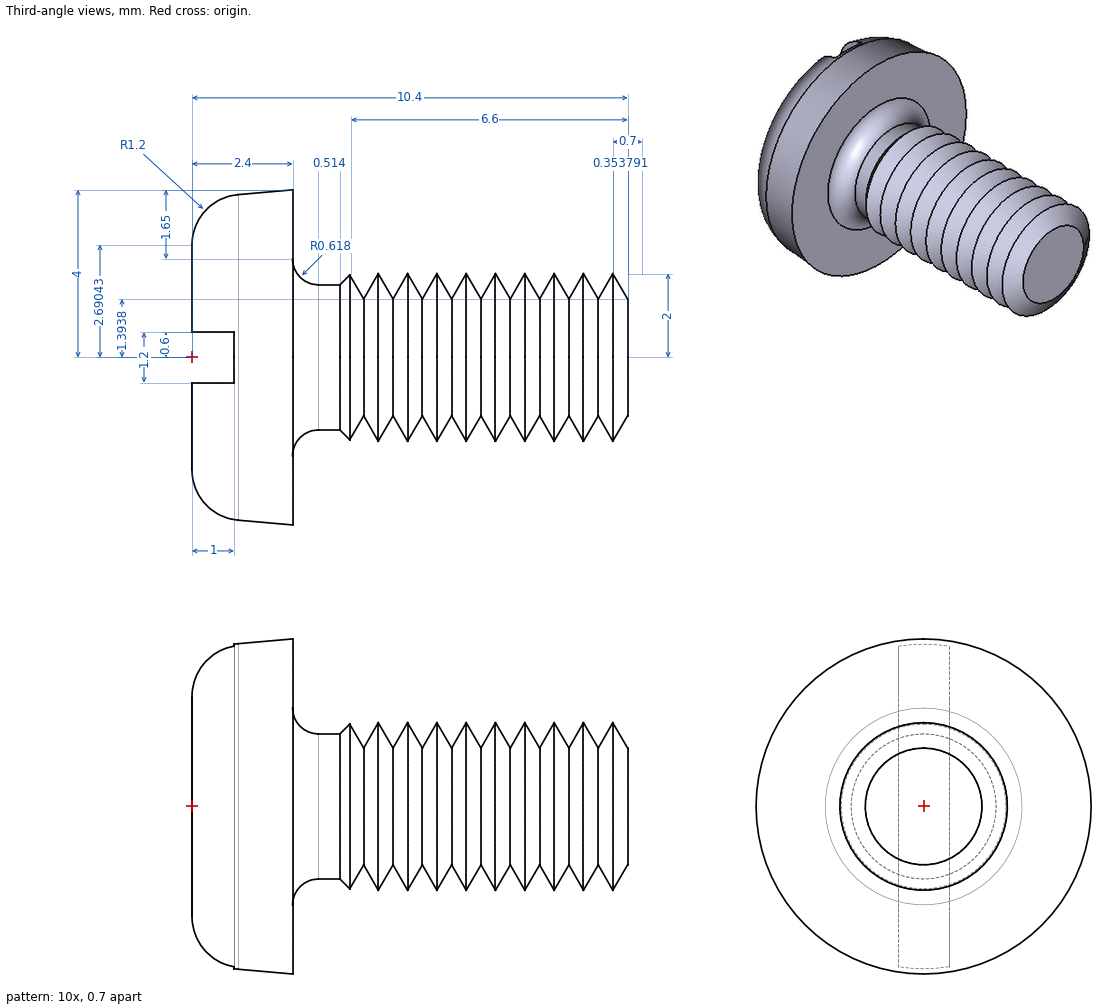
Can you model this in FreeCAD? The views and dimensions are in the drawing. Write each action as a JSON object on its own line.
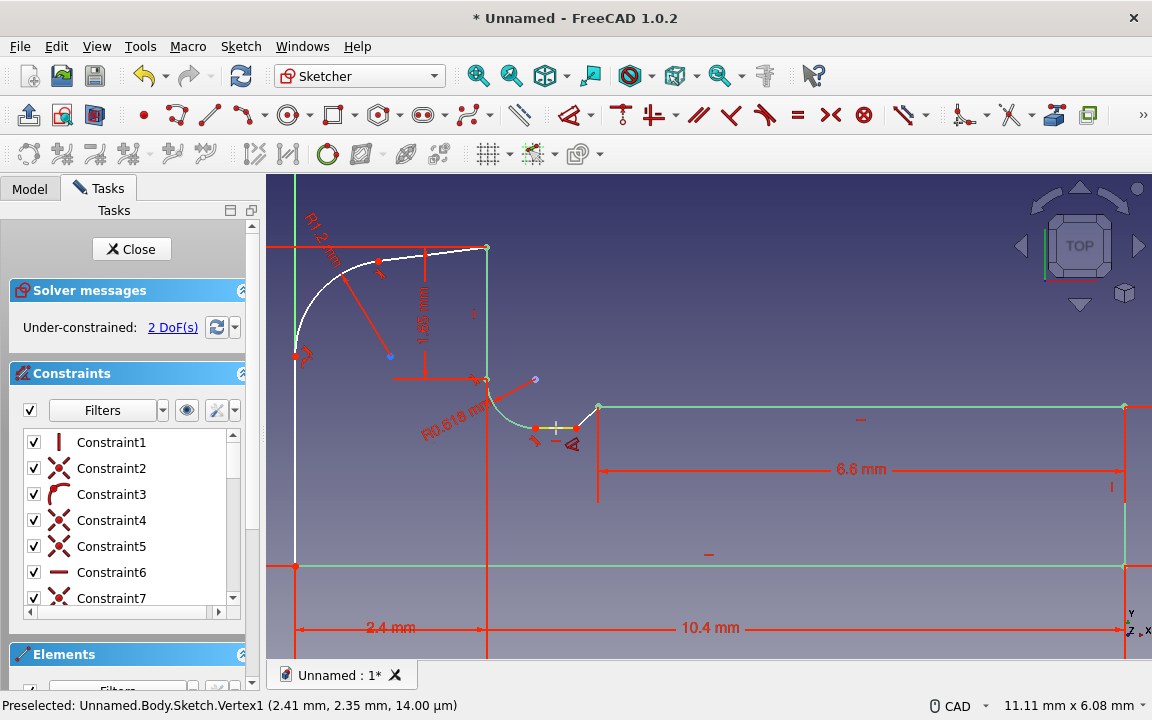
{"action": "left_click", "coordinate": [556, 428]}
{"action": "left_click", "coordinate": [556, 462]}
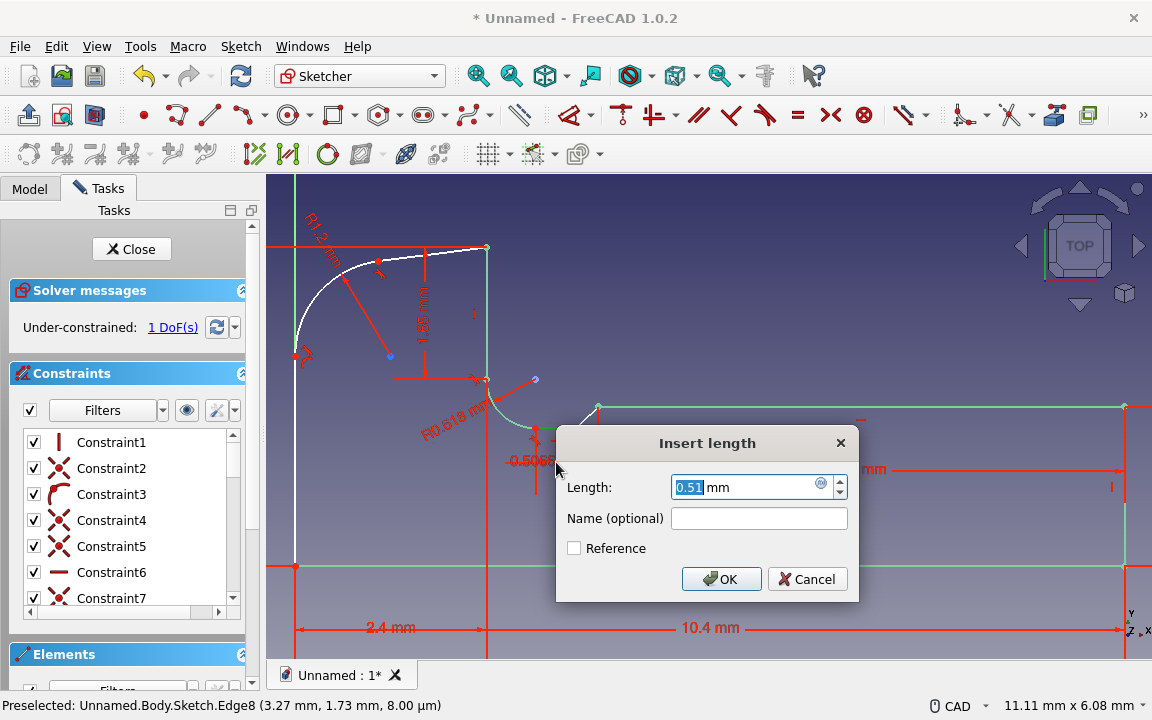
{"action": "type", "text": "0.514"}
{"action": "key", "text": "Return"}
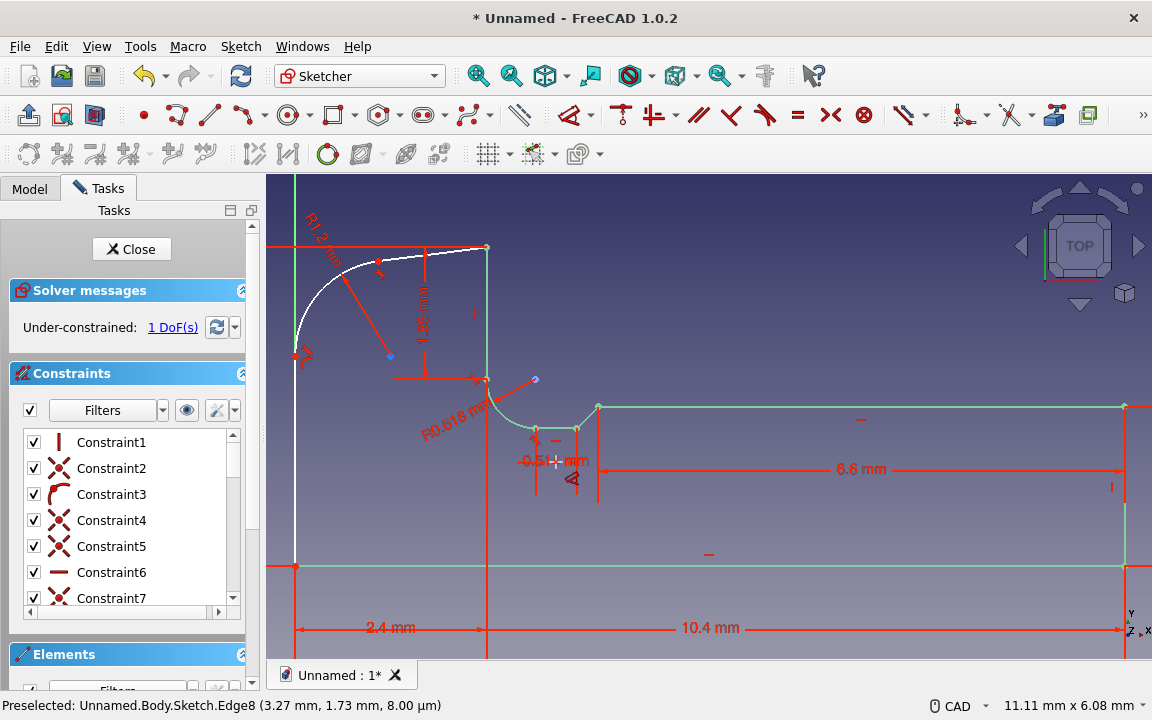
{"action": "left_click", "coordinate": [295, 419]}
{"action": "left_click", "coordinate": [329, 461]}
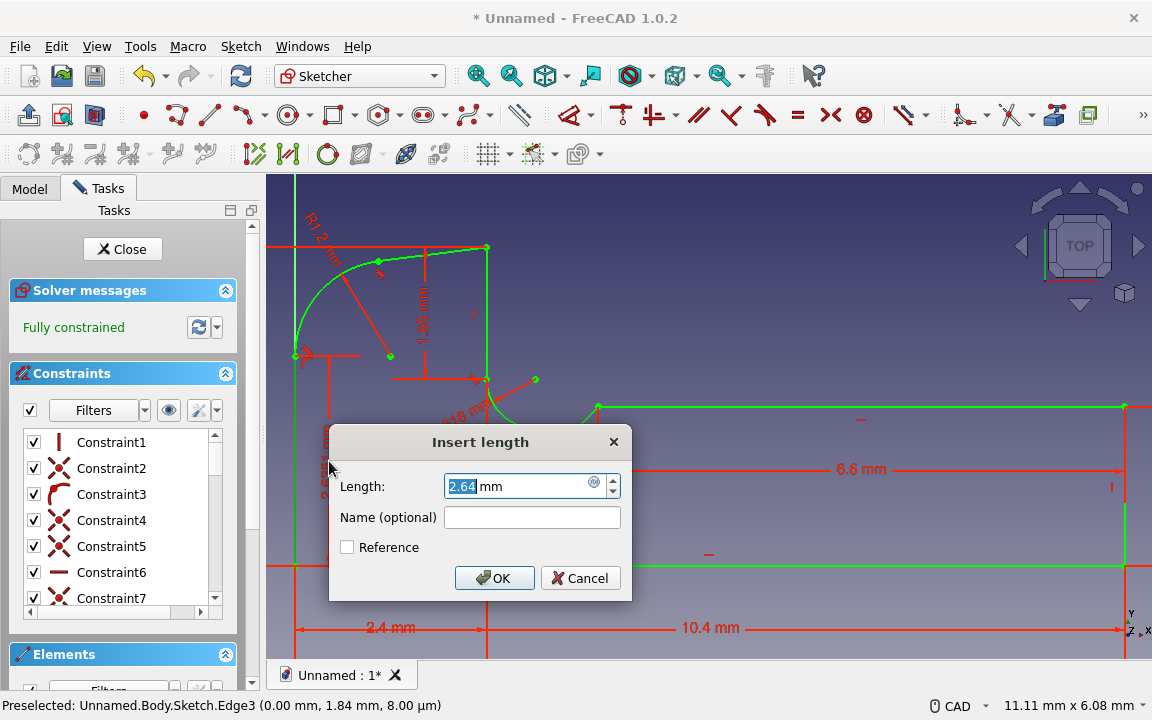
{"action": "type", "text": "2.69043"}
{"action": "key", "text": "Return"}
{"action": "key", "text": "Escape"}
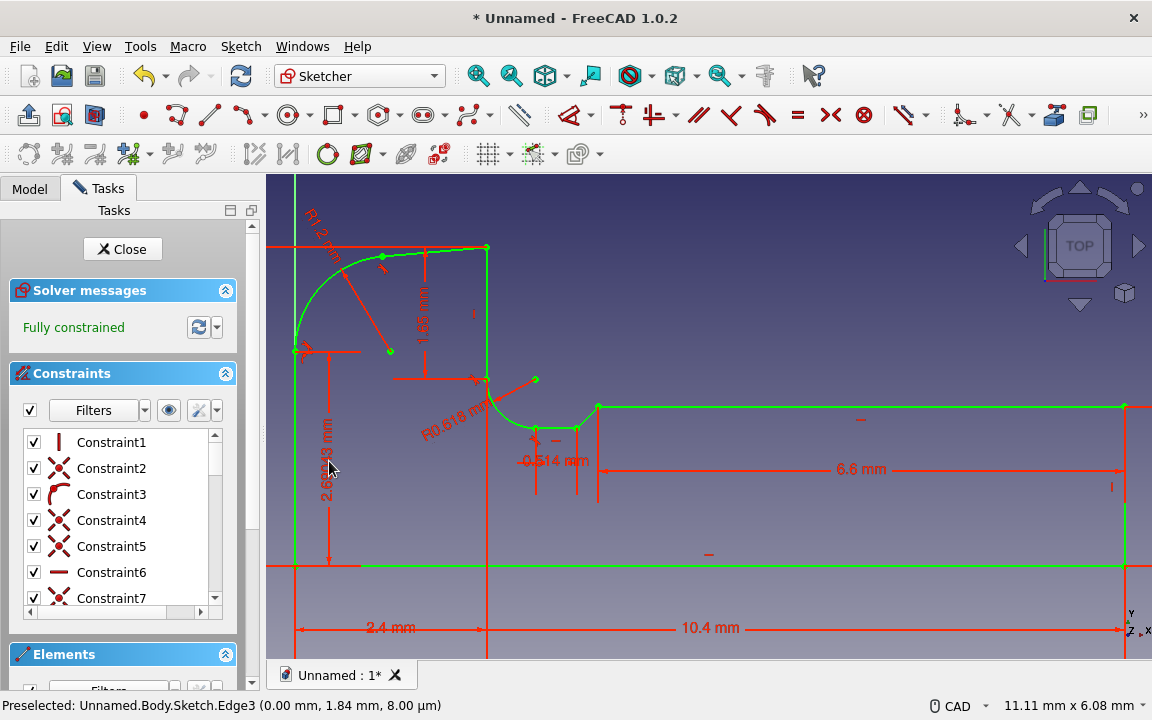
{"action": "left_click", "coordinate": [123, 249]}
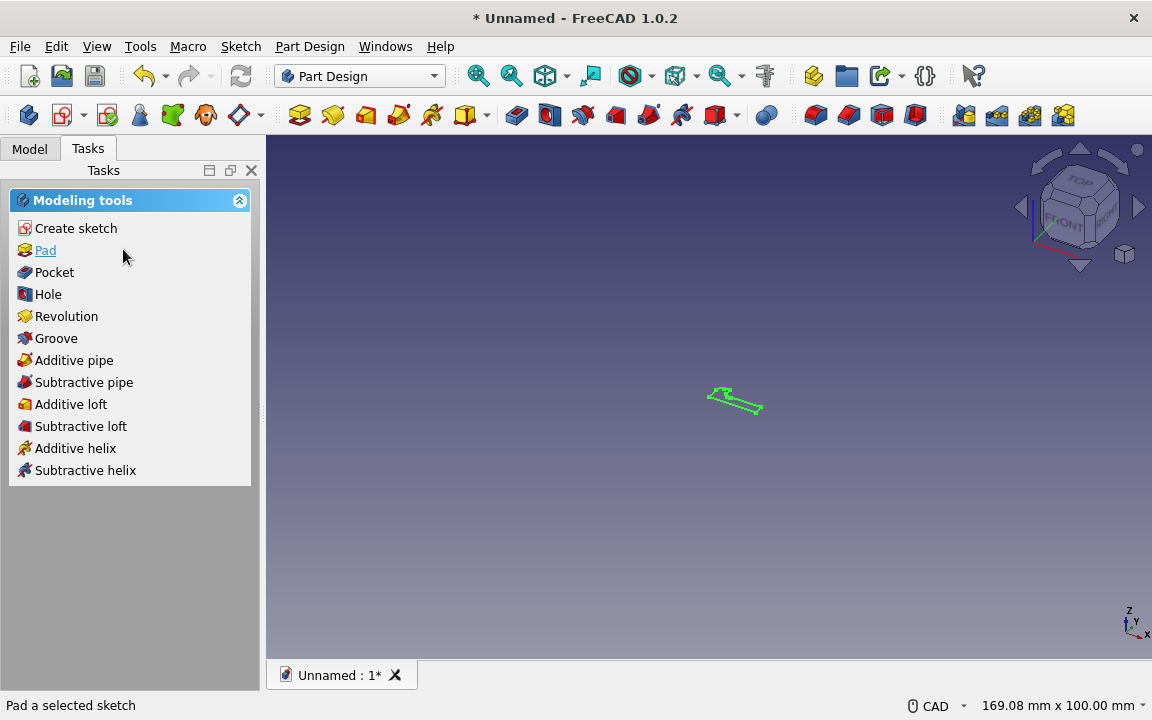
{"action": "left_click", "coordinate": [333, 116]}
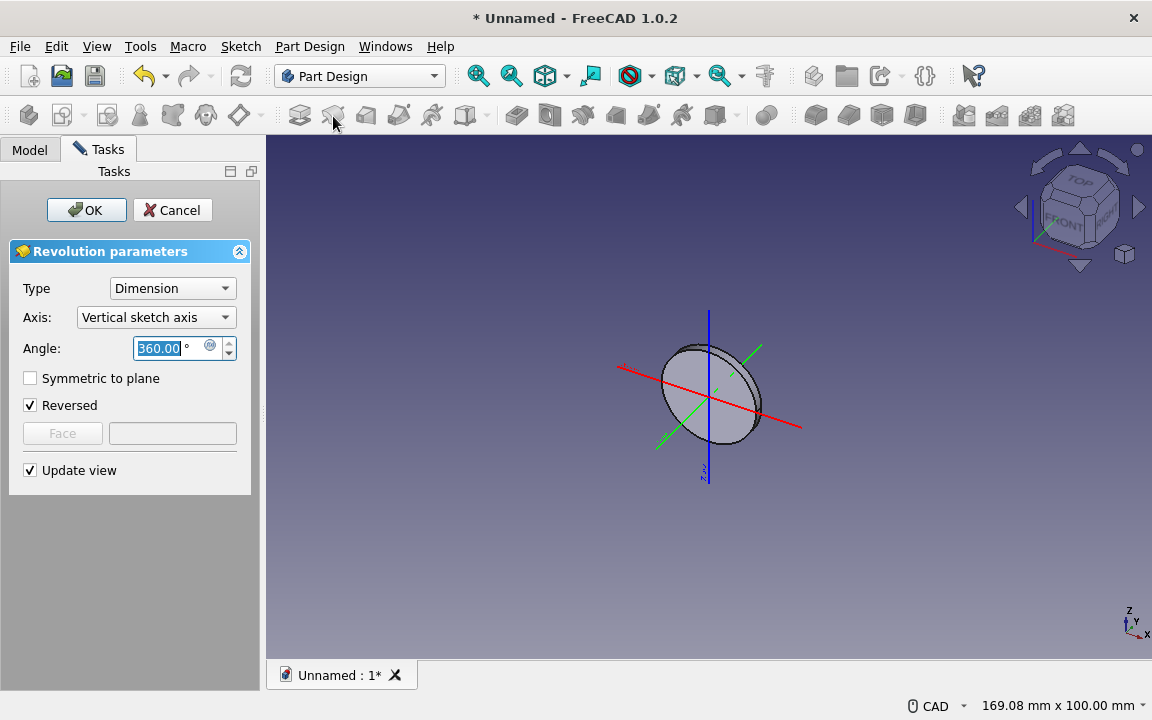
{"action": "left_click", "coordinate": [157, 318]}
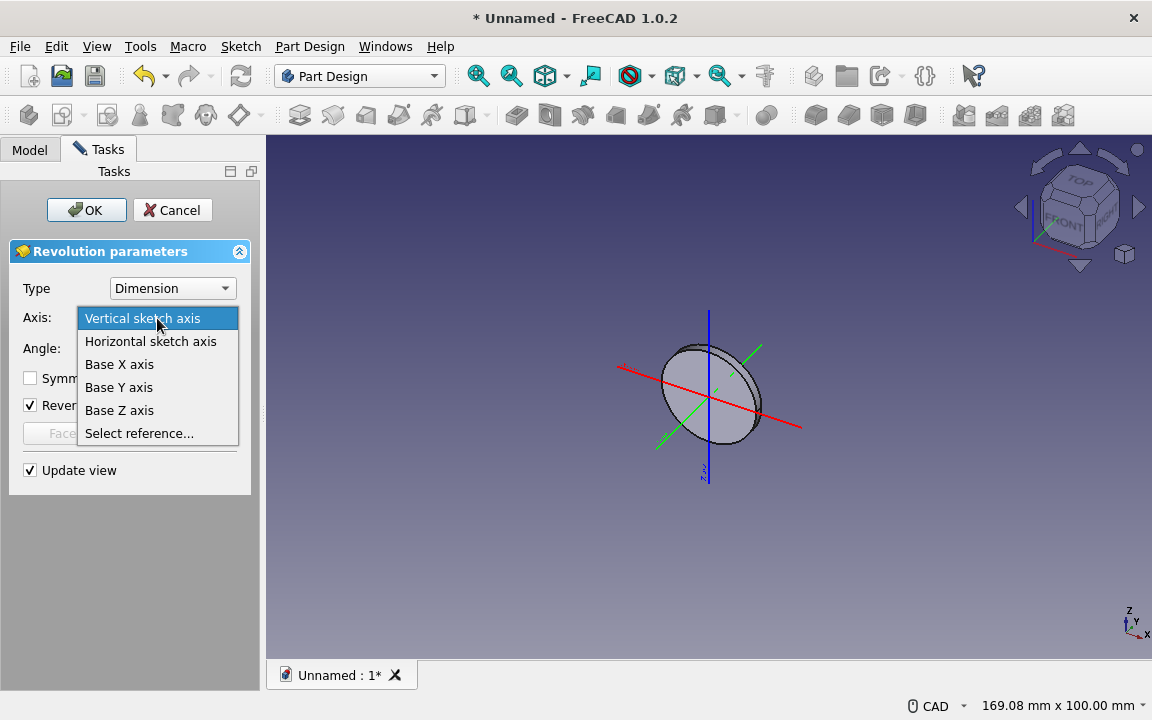
{"action": "left_click", "coordinate": [156, 342]}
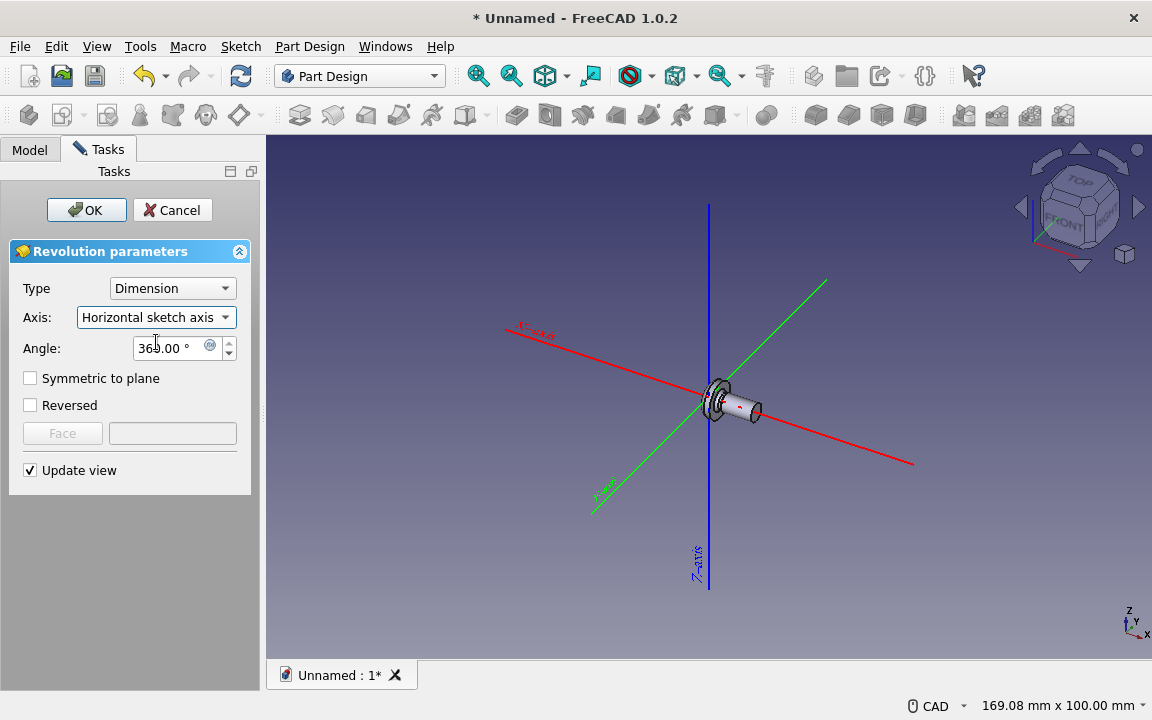
{"action": "left_click", "coordinate": [87, 210]}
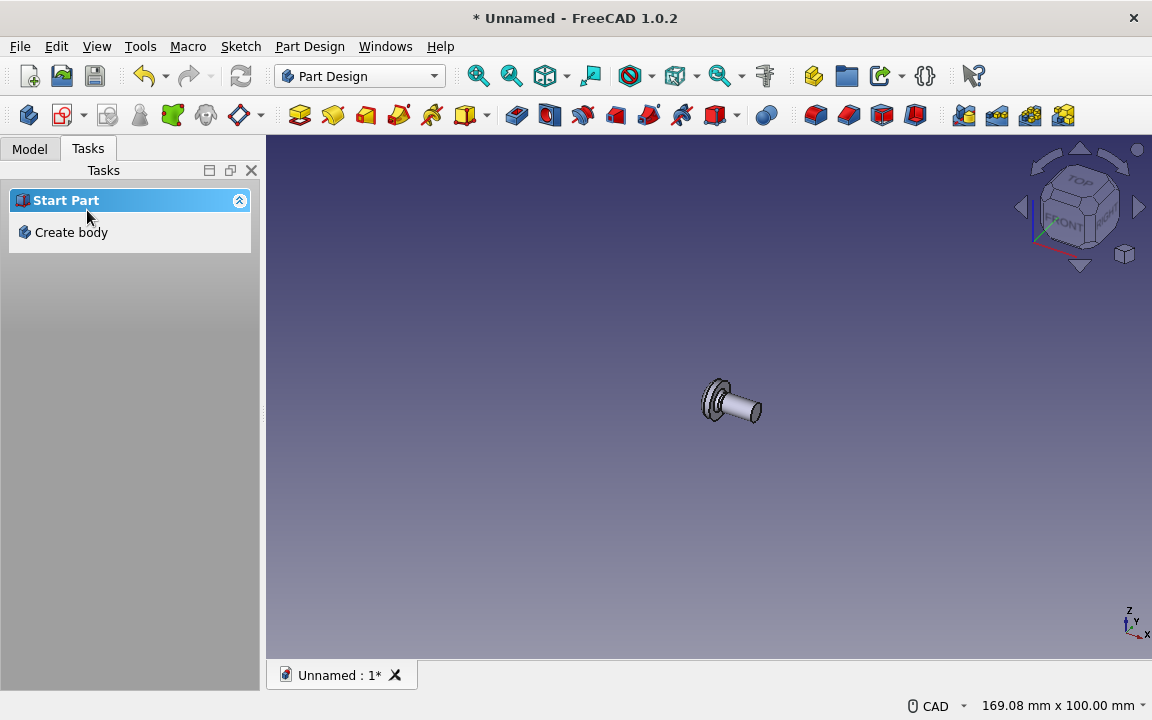
{"action": "left_click", "coordinate": [479, 76]}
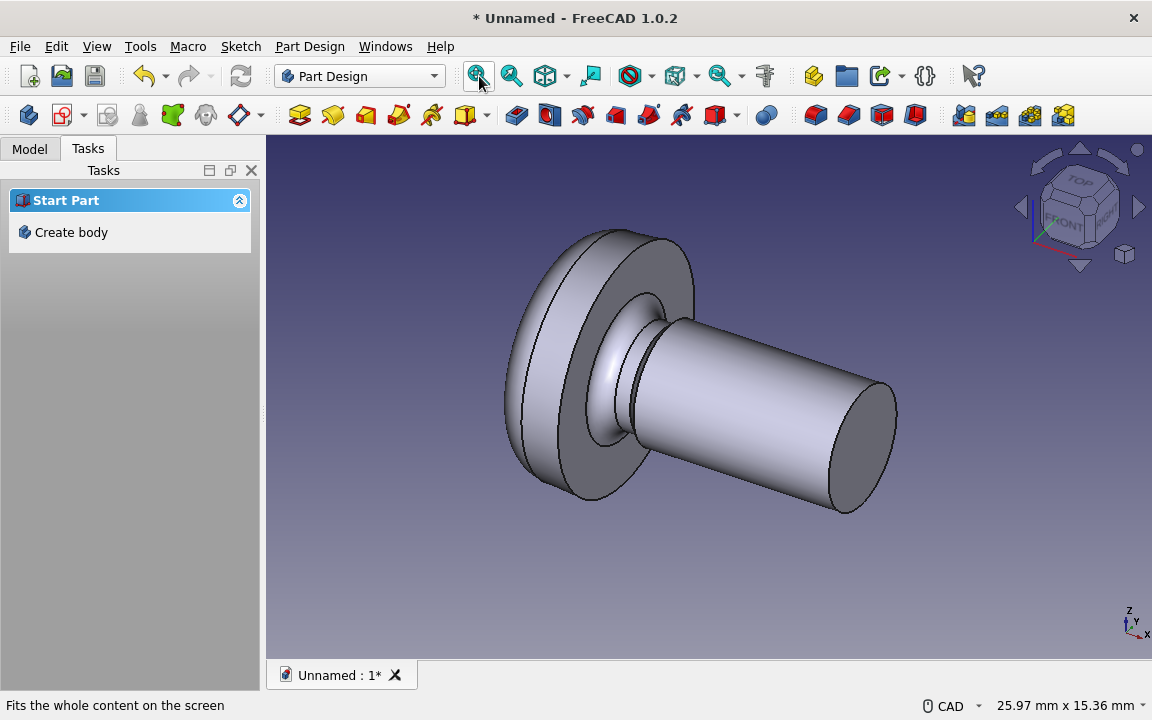
{"action": "left_click", "coordinate": [62, 116]}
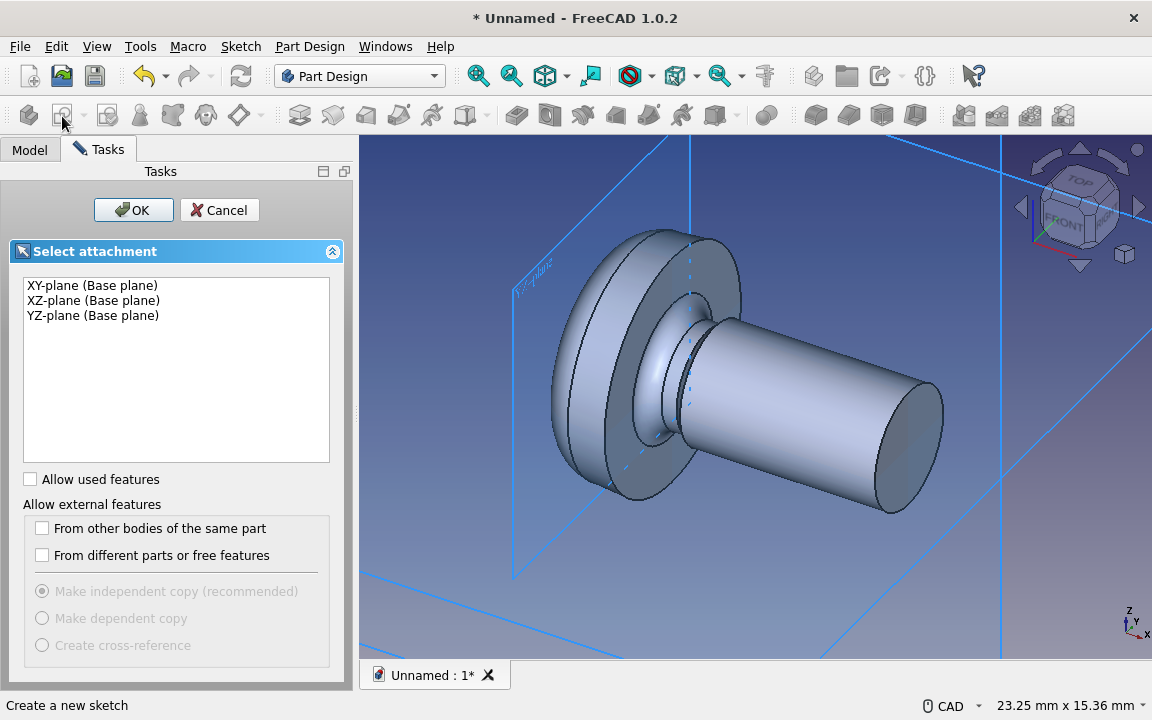
{"action": "left_click", "coordinate": [84, 286]}